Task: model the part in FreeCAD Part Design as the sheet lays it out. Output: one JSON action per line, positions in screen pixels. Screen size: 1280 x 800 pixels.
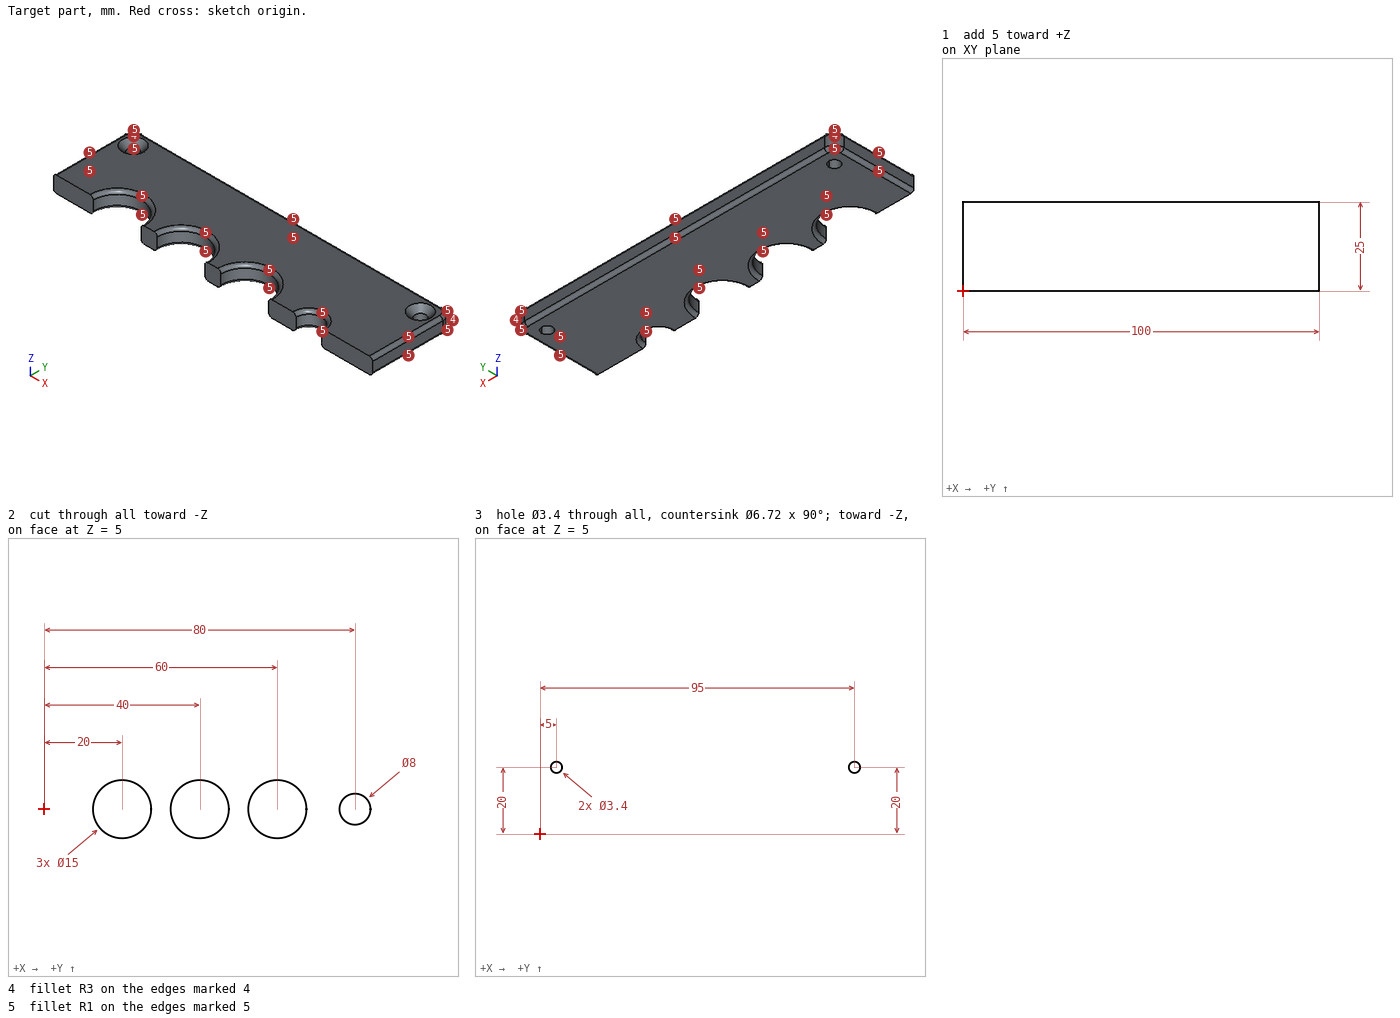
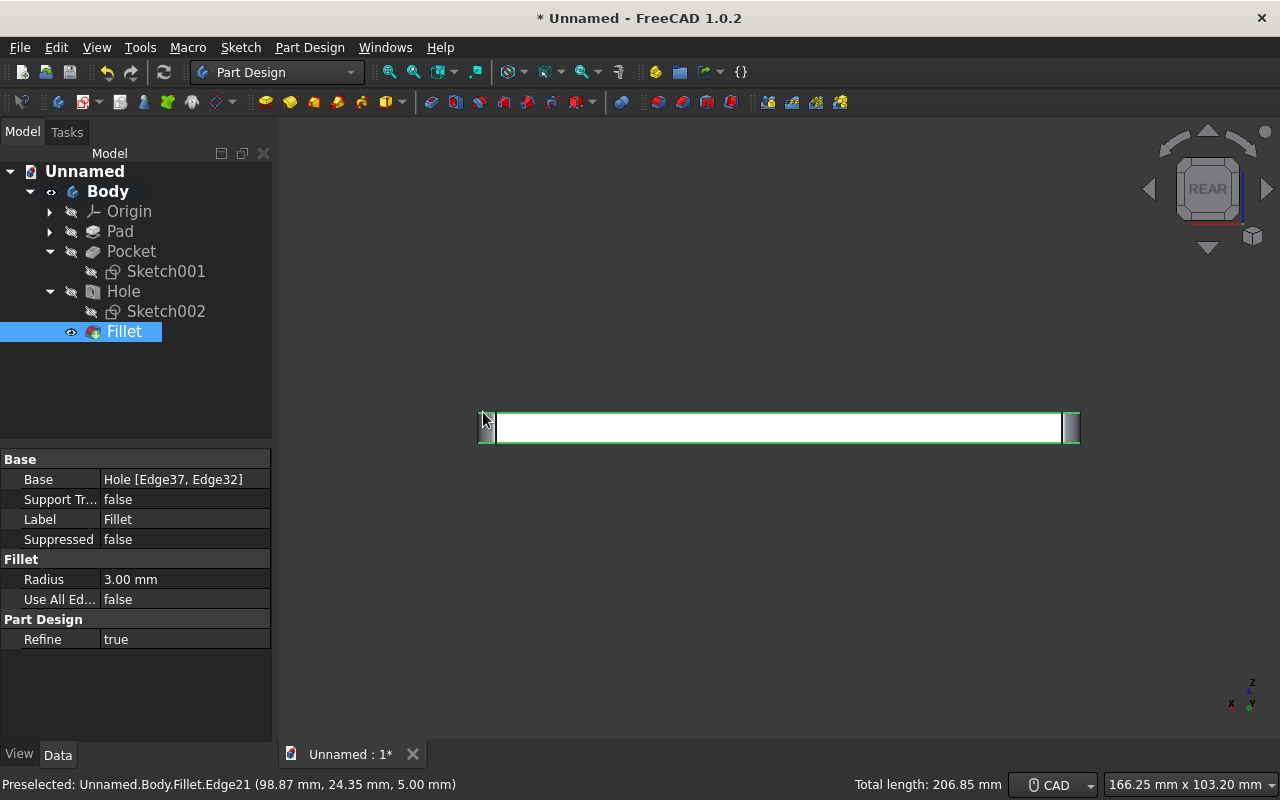
{"action": "key", "text": "0"}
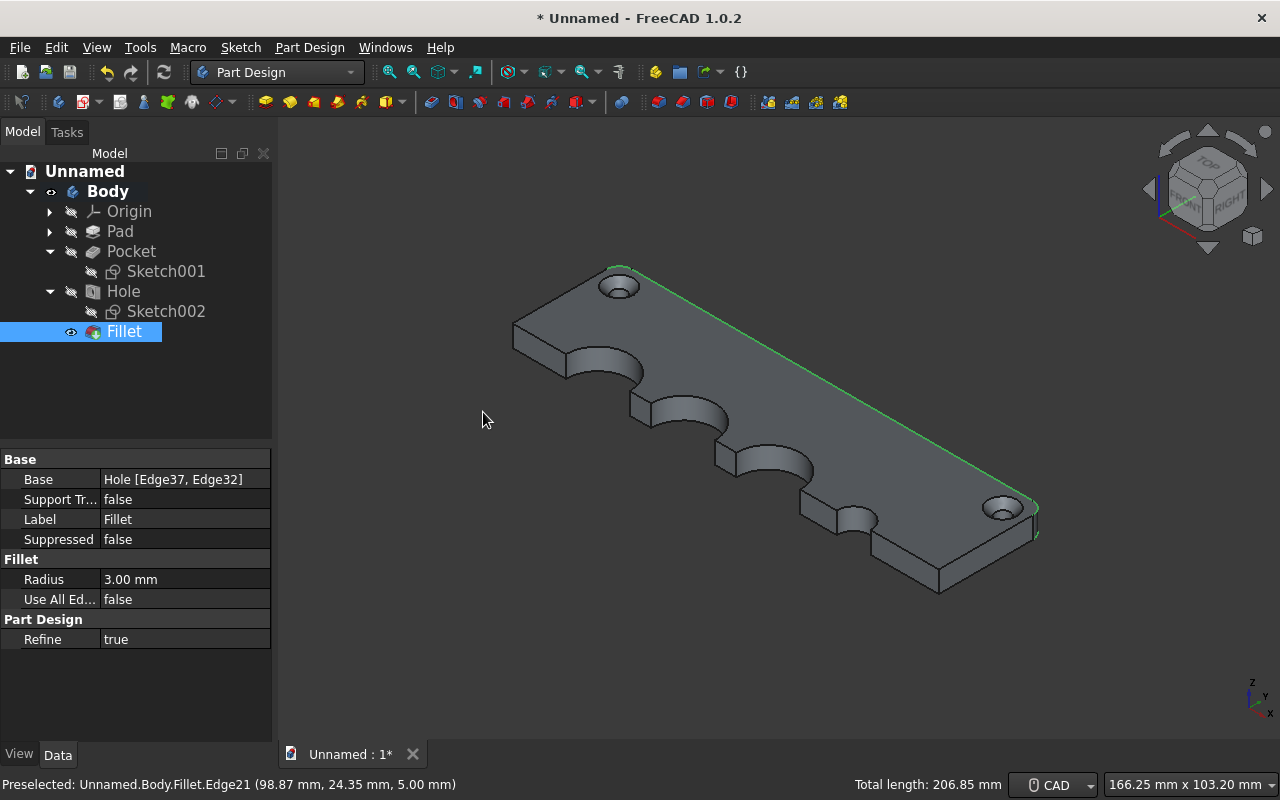
{"action": "left_click", "coordinate": [986, 541], "text": "ctrl"}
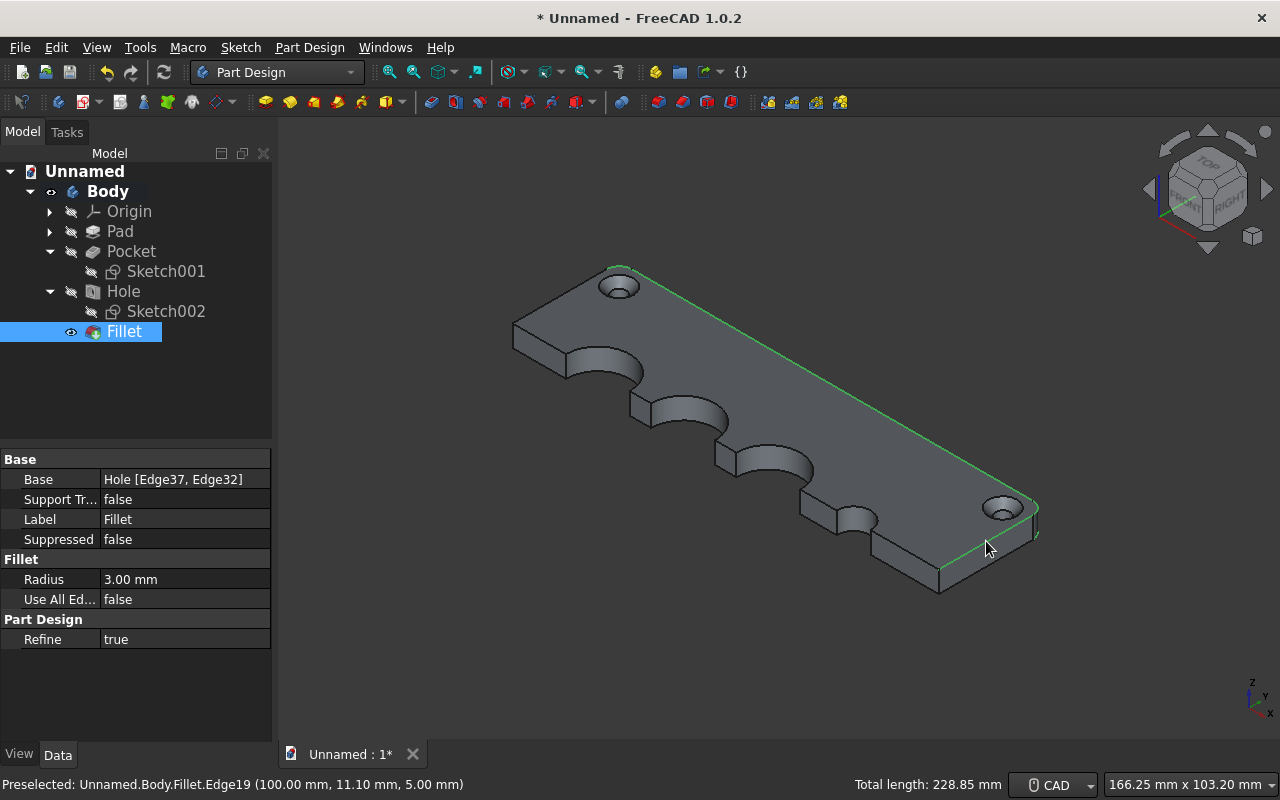
{"action": "left_click", "coordinate": [630, 353], "text": "ctrl"}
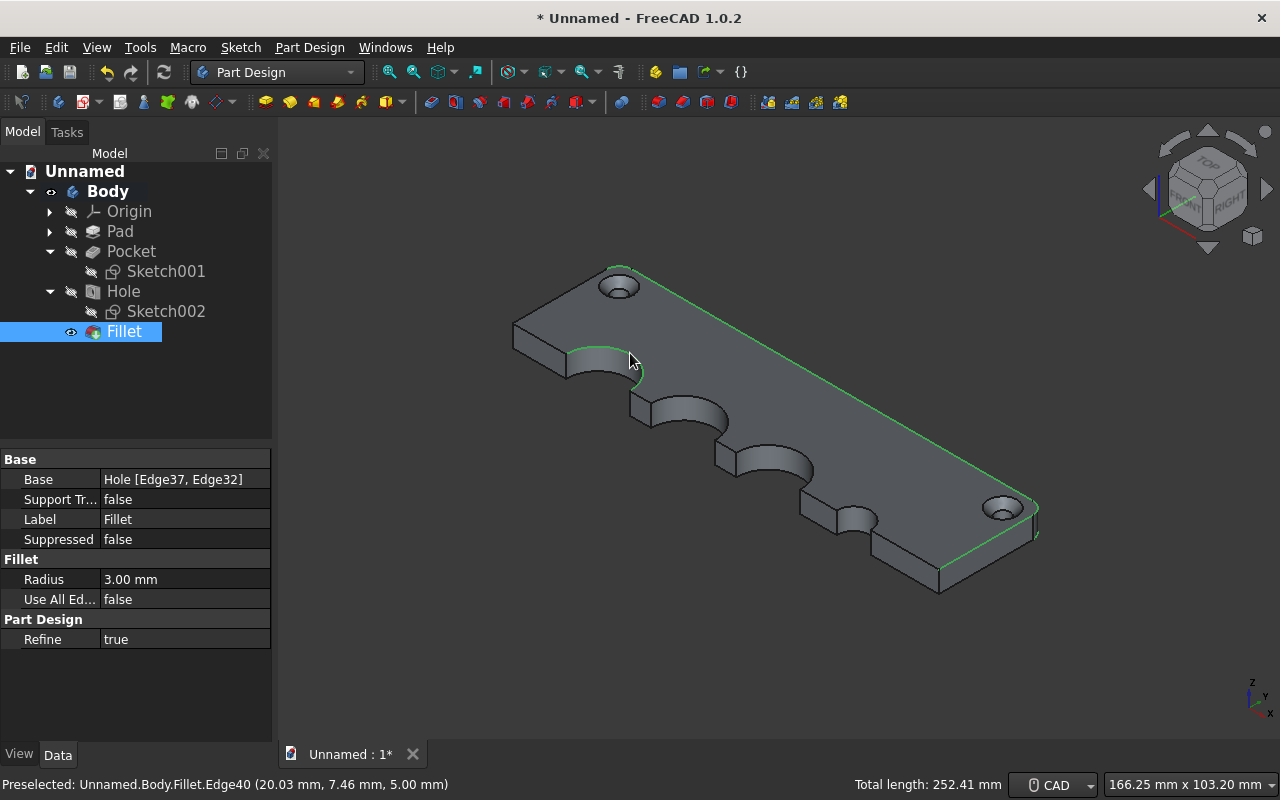
{"action": "left_click", "coordinate": [715, 402], "text": "ctrl"}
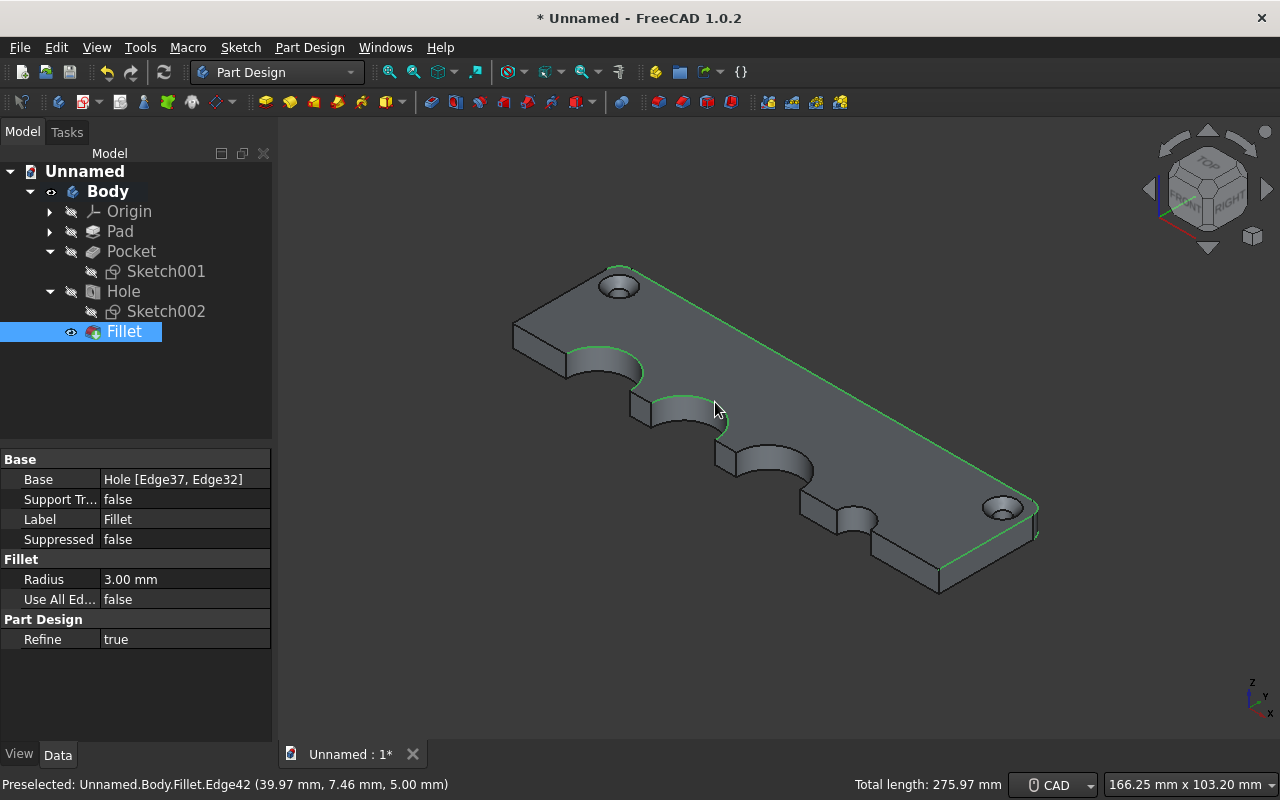
{"action": "left_click", "coordinate": [800, 452], "text": "ctrl"}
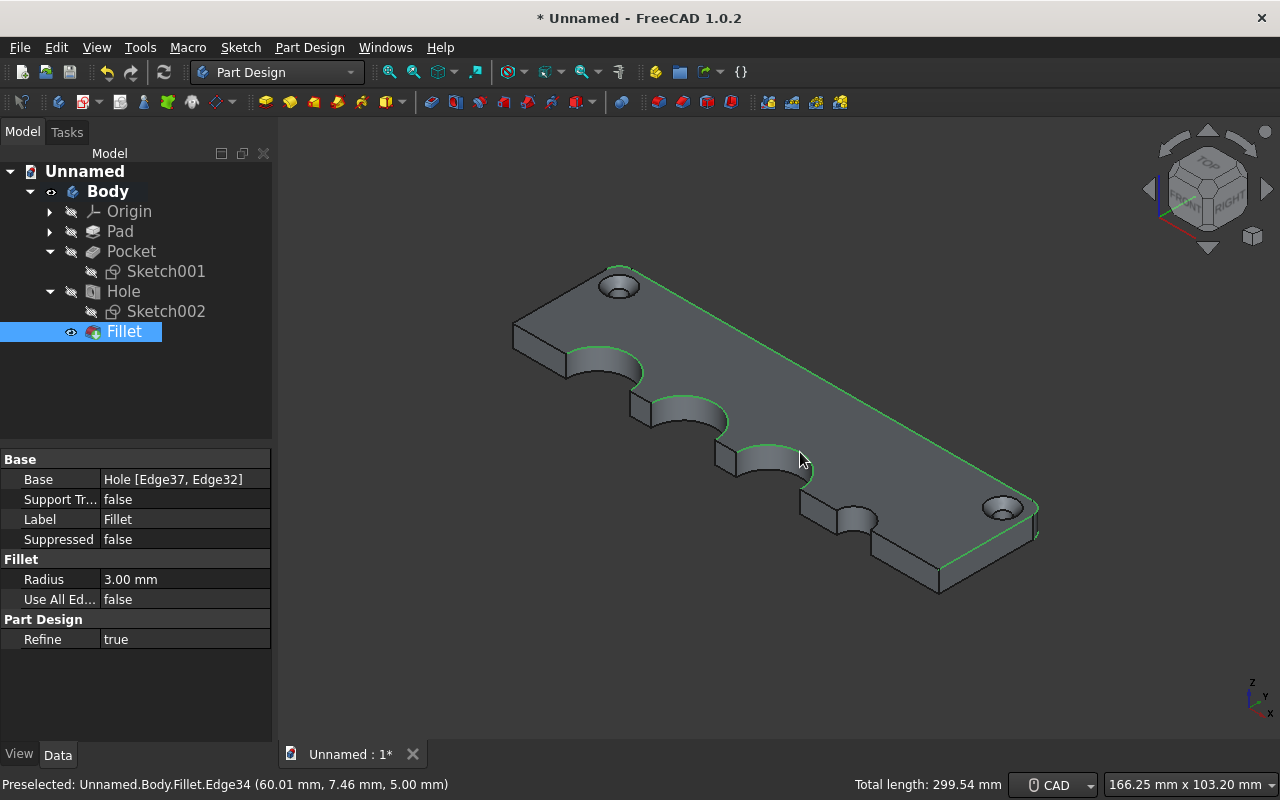
{"action": "left_click", "coordinate": [871, 509], "text": "ctrl"}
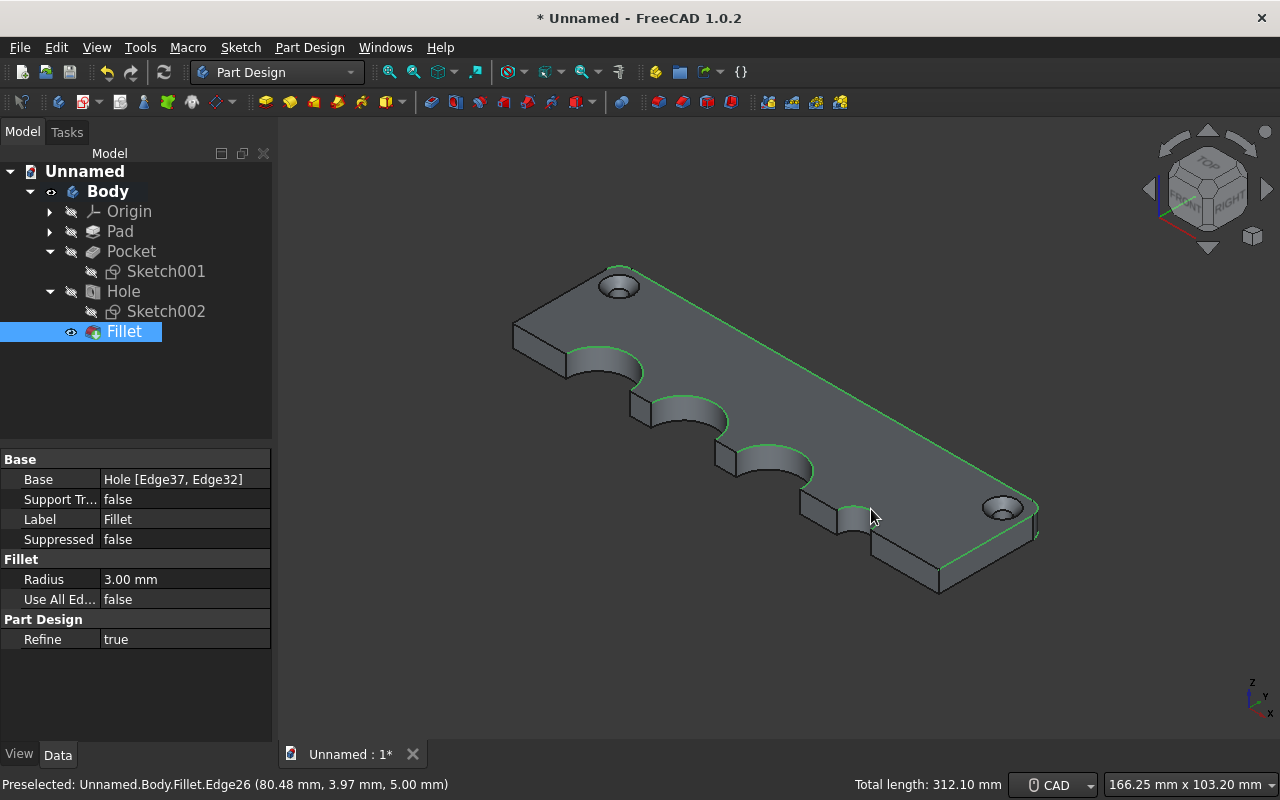
{"action": "key", "text": "2"}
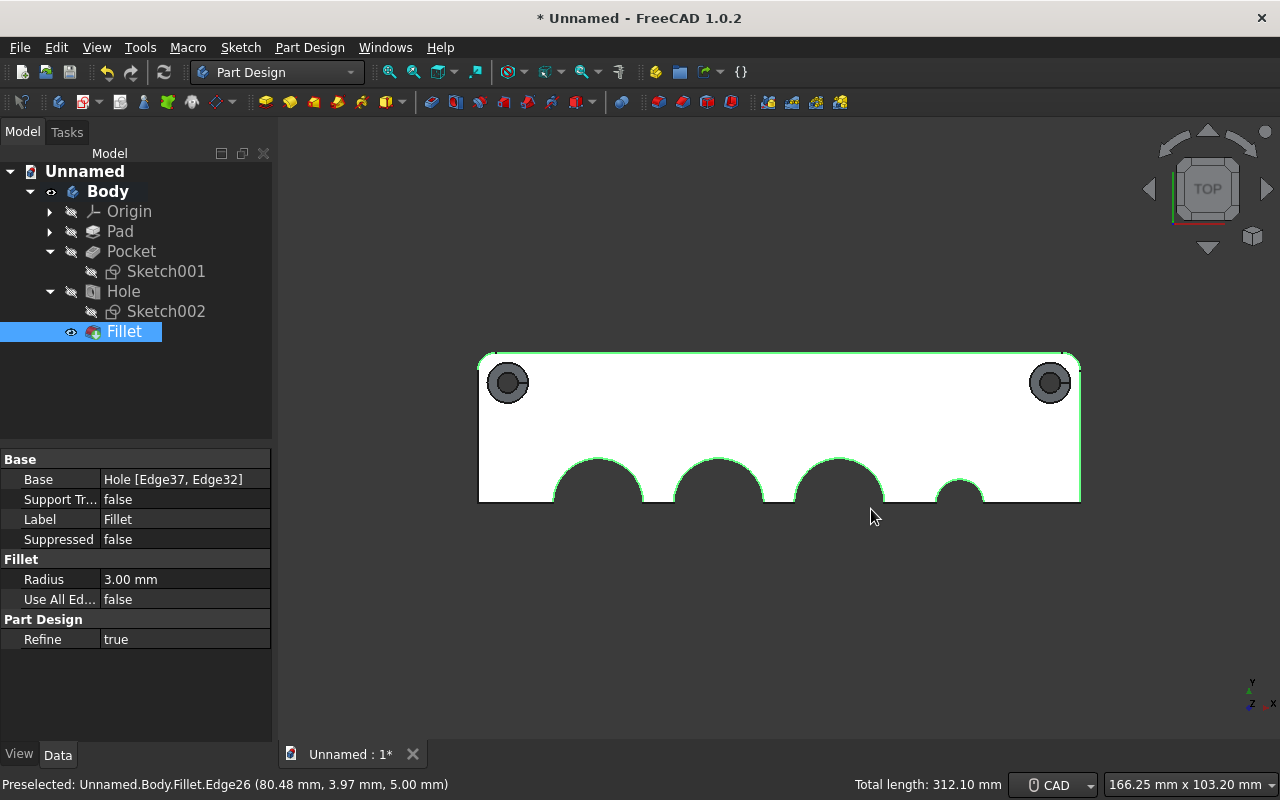
{"action": "left_click", "coordinate": [478, 436], "text": "ctrl"}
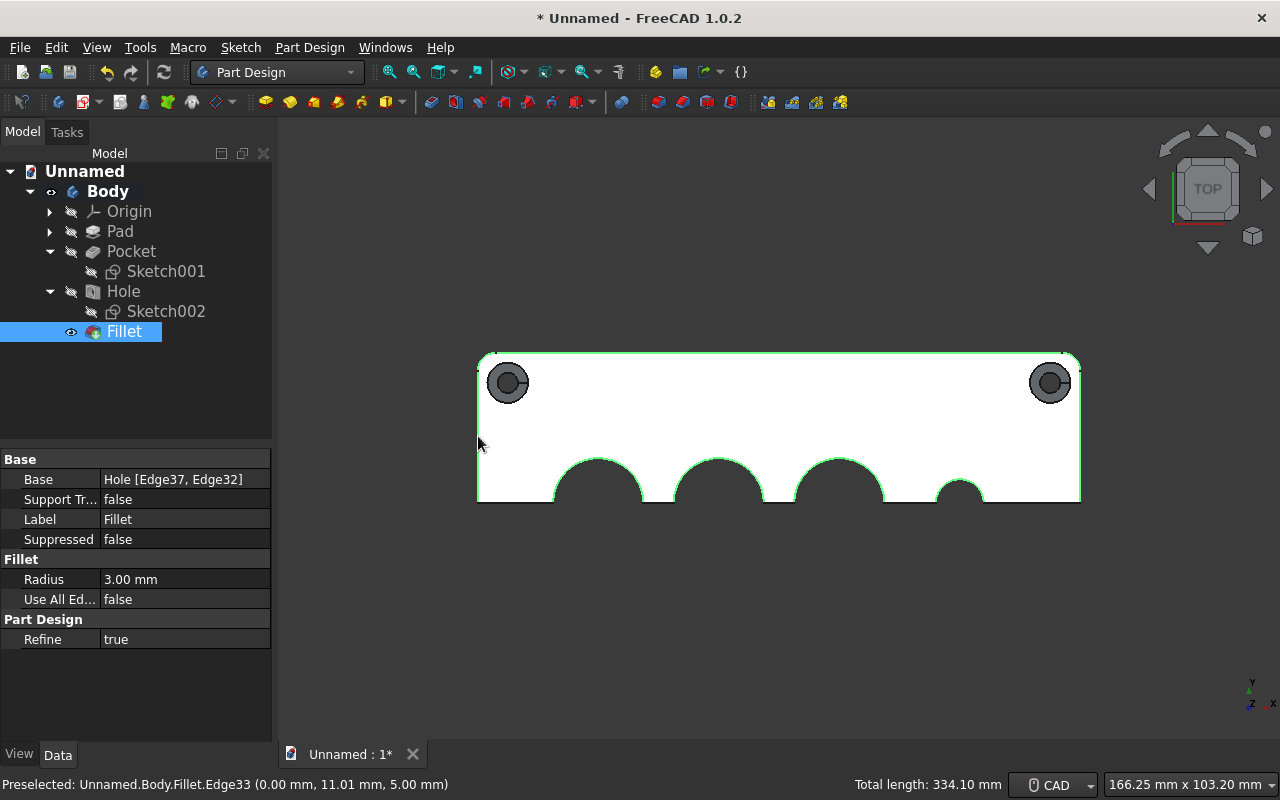
{"action": "key", "text": "1"}